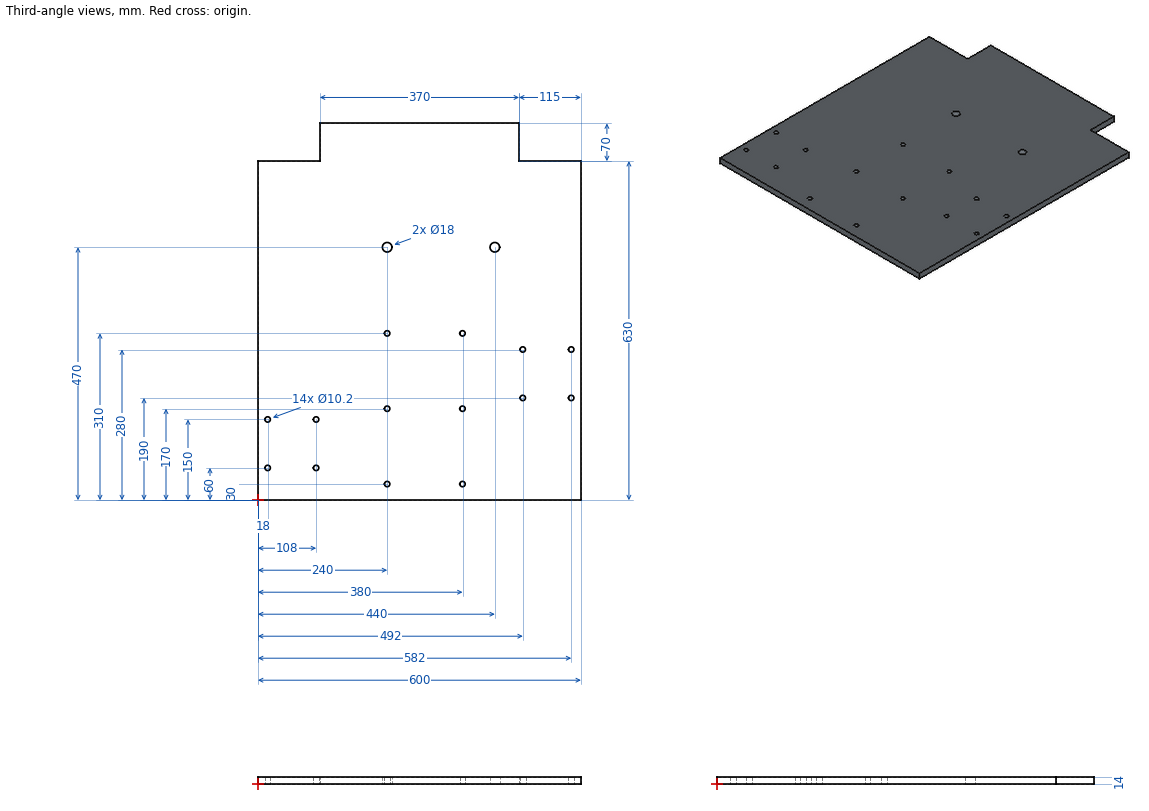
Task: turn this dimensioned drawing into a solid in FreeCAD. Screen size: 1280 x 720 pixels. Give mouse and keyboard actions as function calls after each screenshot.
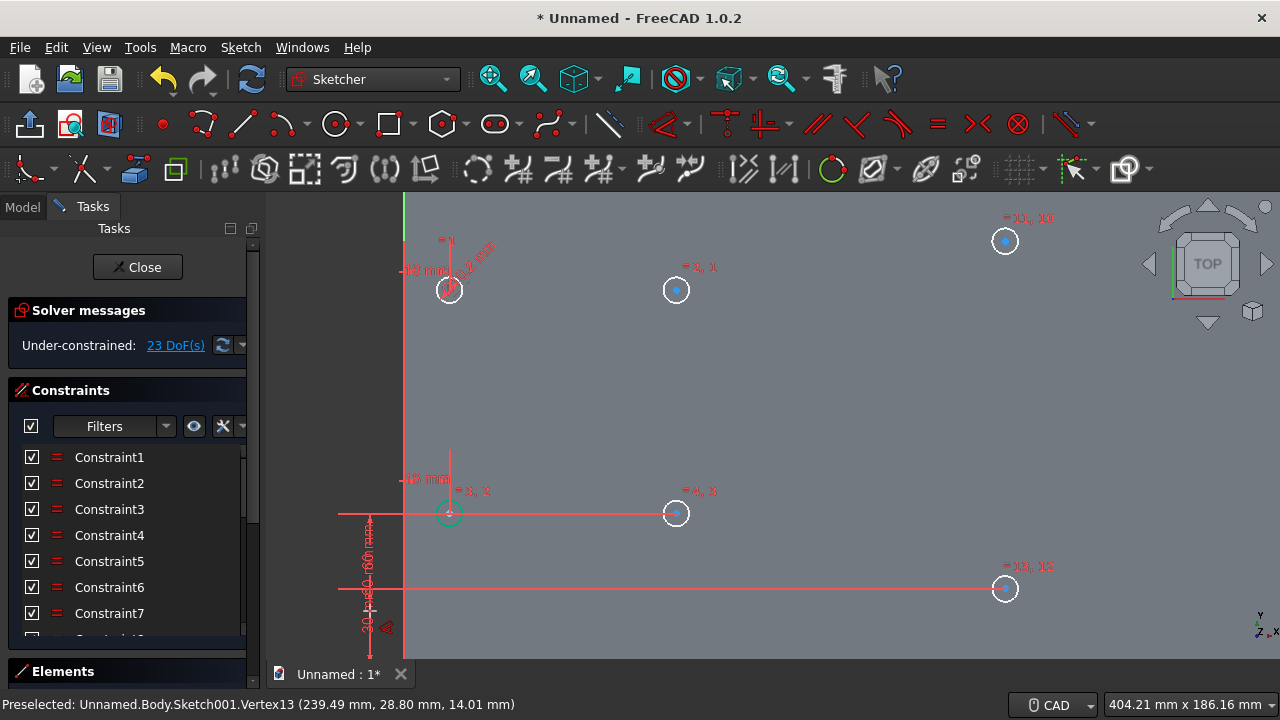
scroll(451, 517, down, 5)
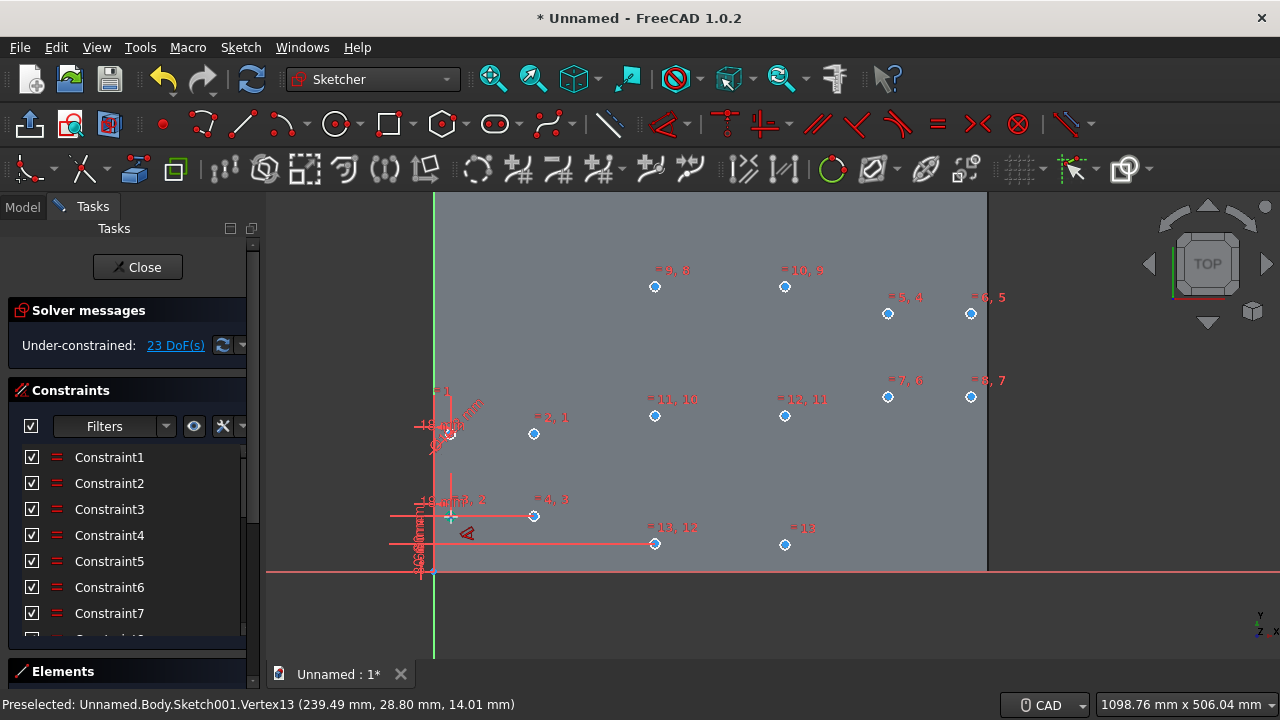
scroll(785, 545, up, 2)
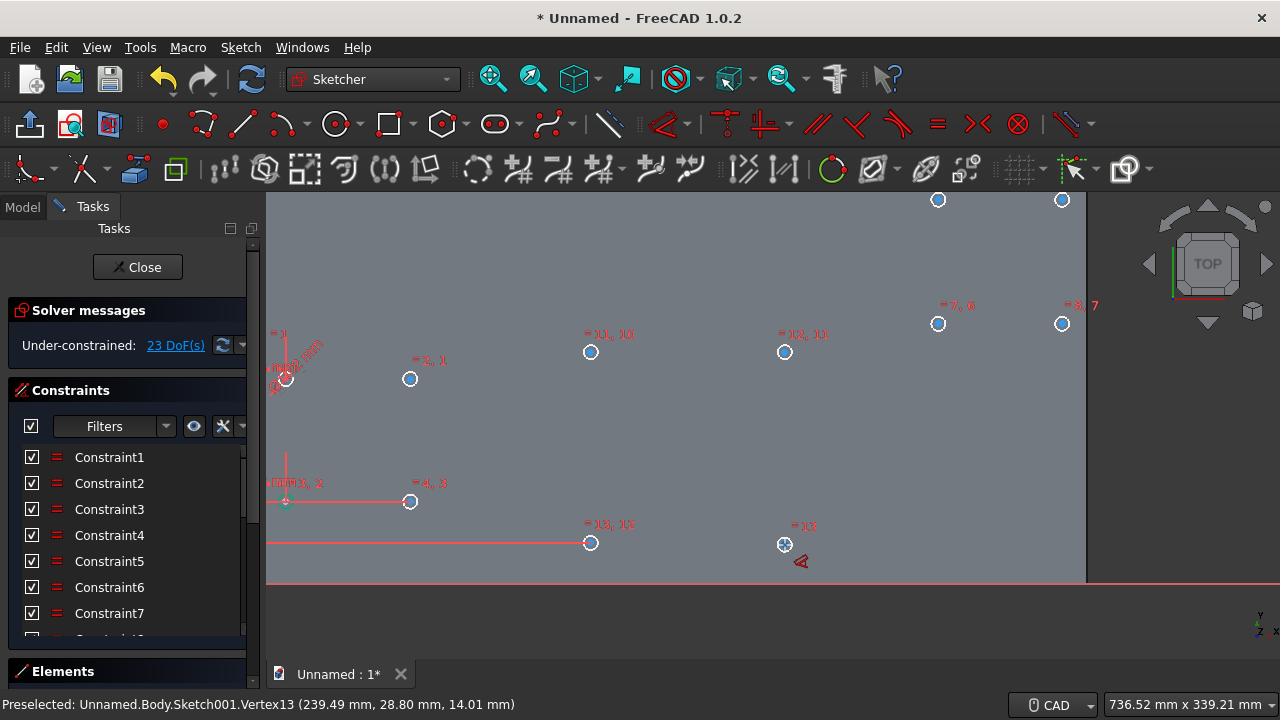
click(785, 545)
click(819, 564)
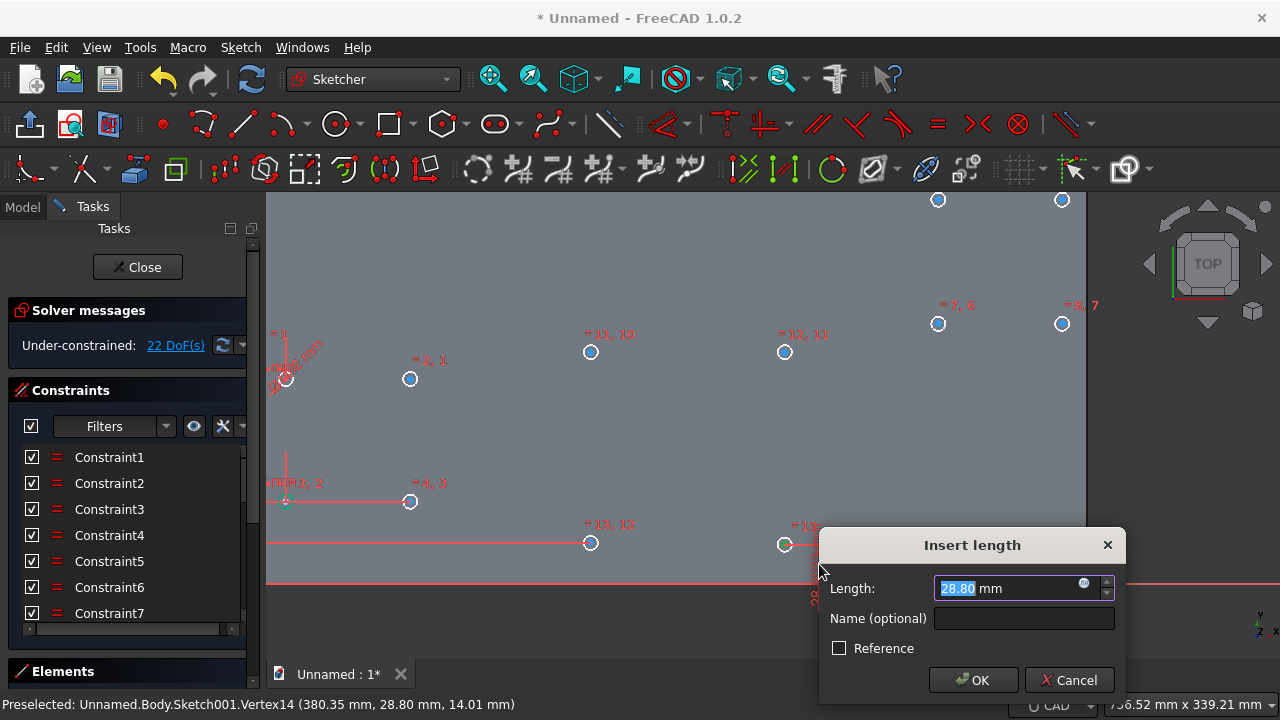
text(30)
key(Return)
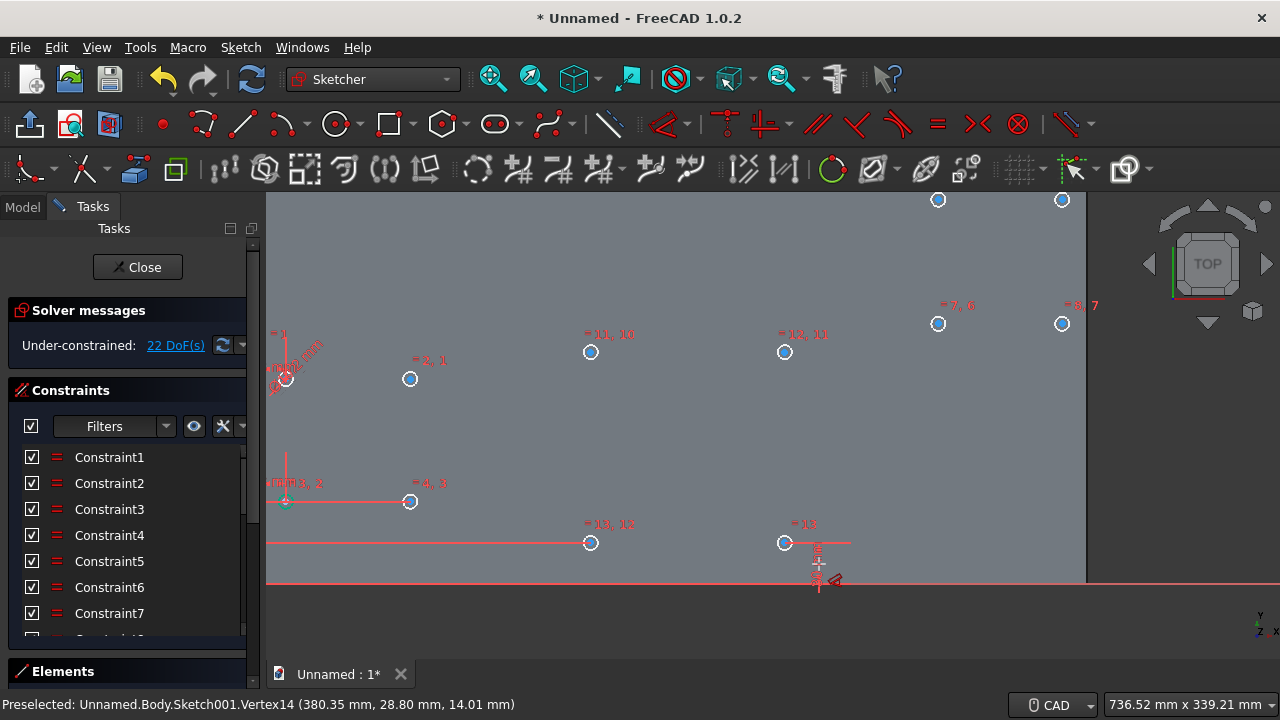
scroll(784, 544, down, 2)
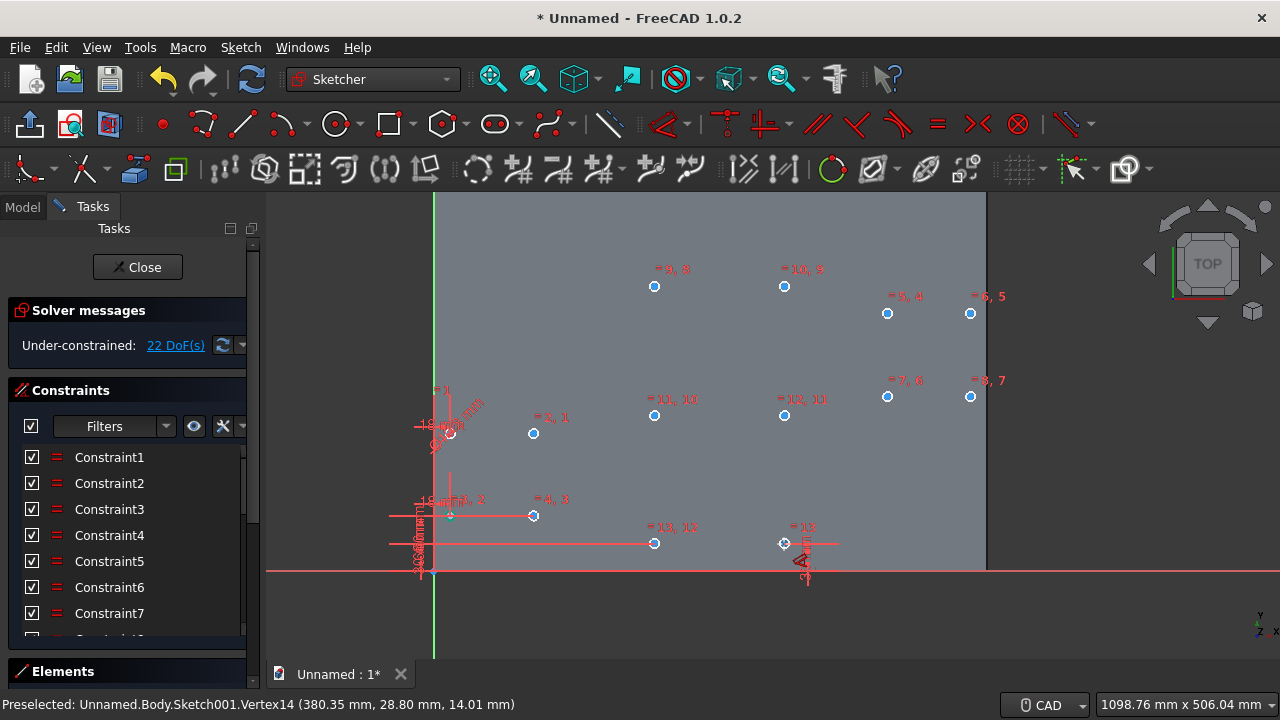
click(450, 434)
click(400, 471)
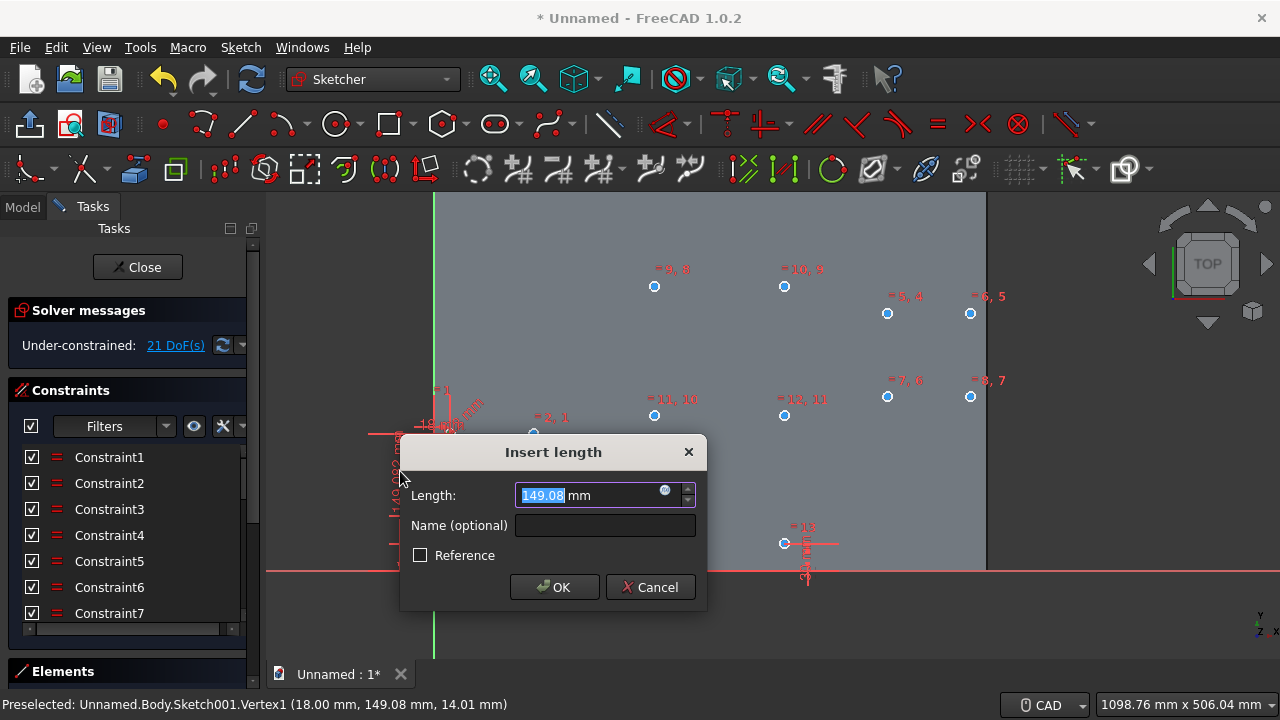
text(150)
key(Return)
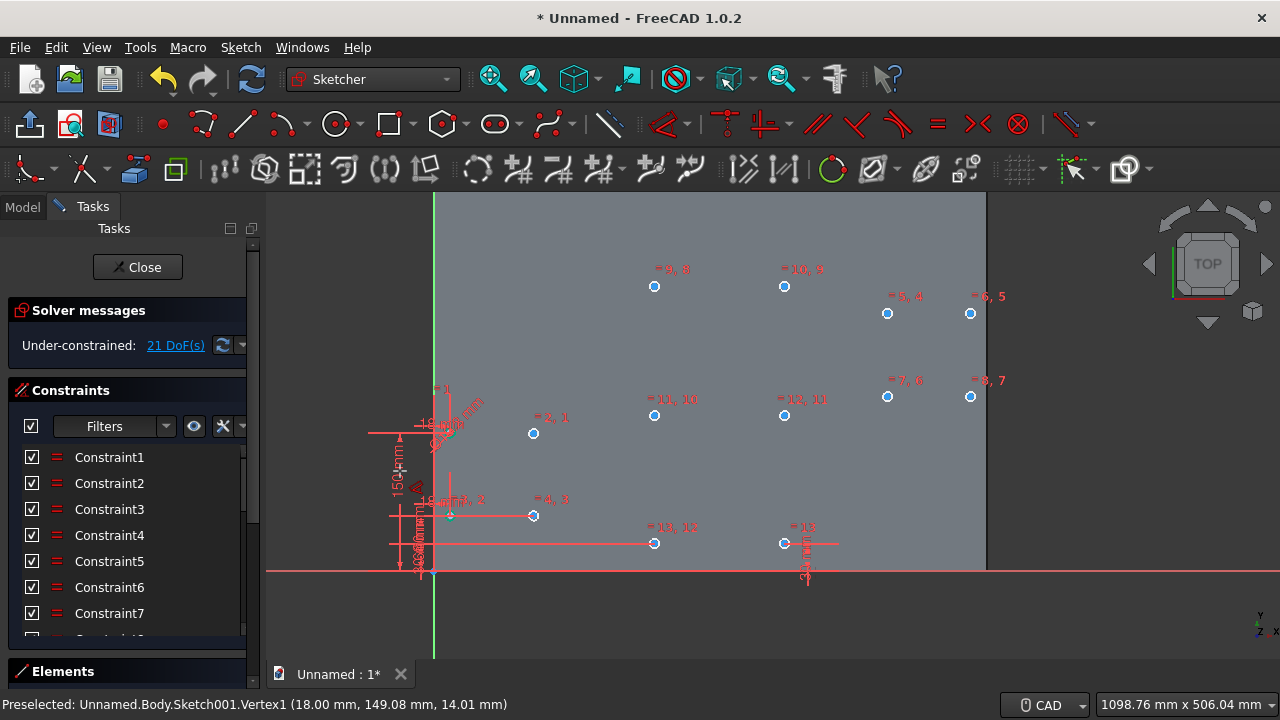
click(534, 434)
click(484, 605)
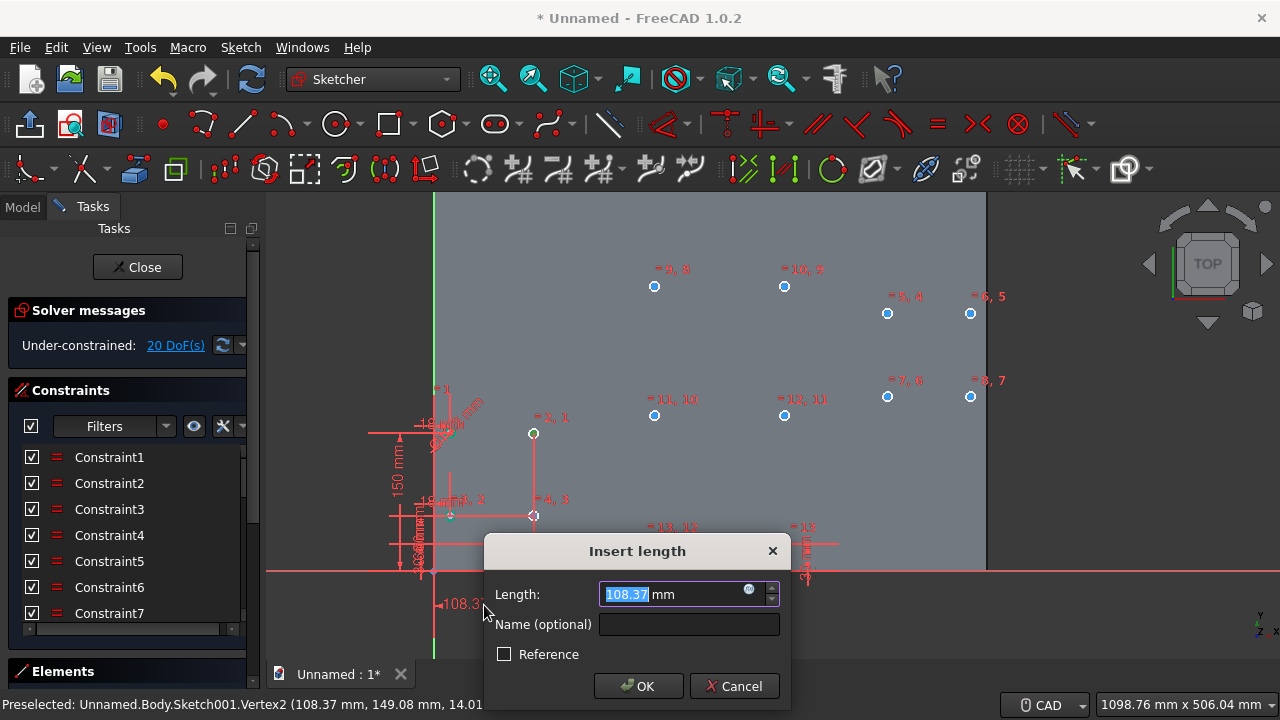
text(108)
key(Return)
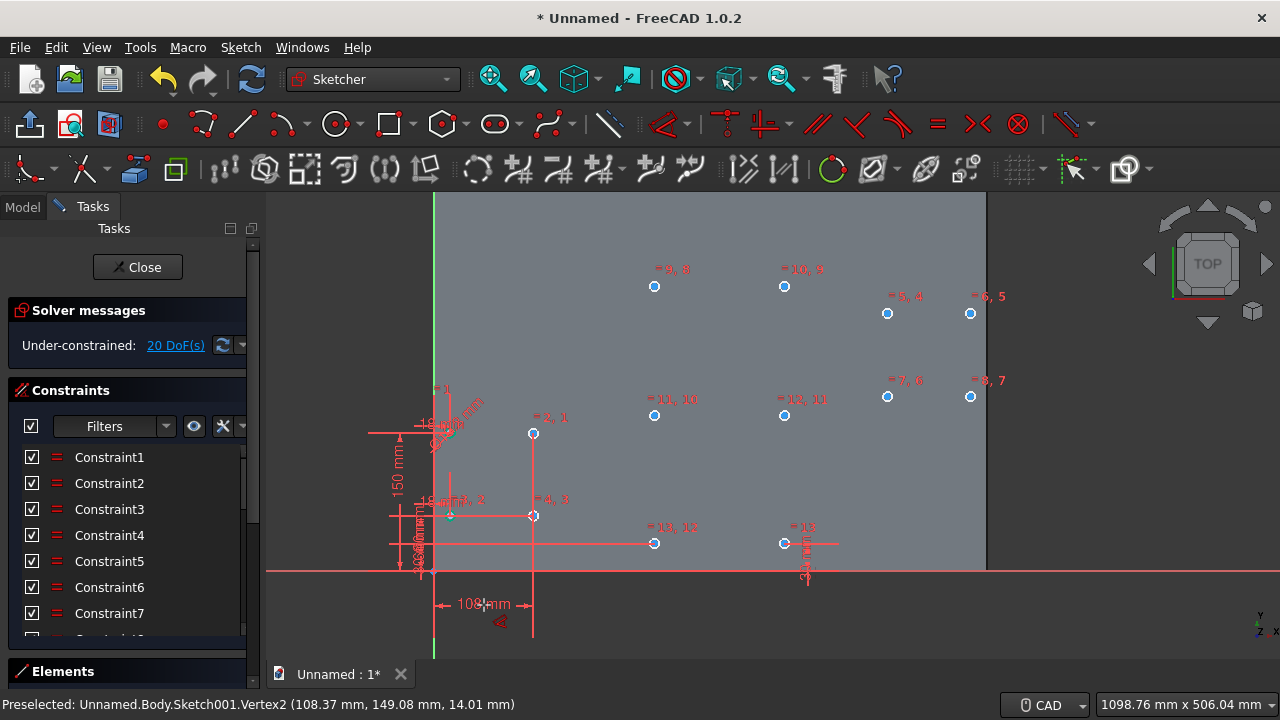
click(533, 434)
click(567, 502)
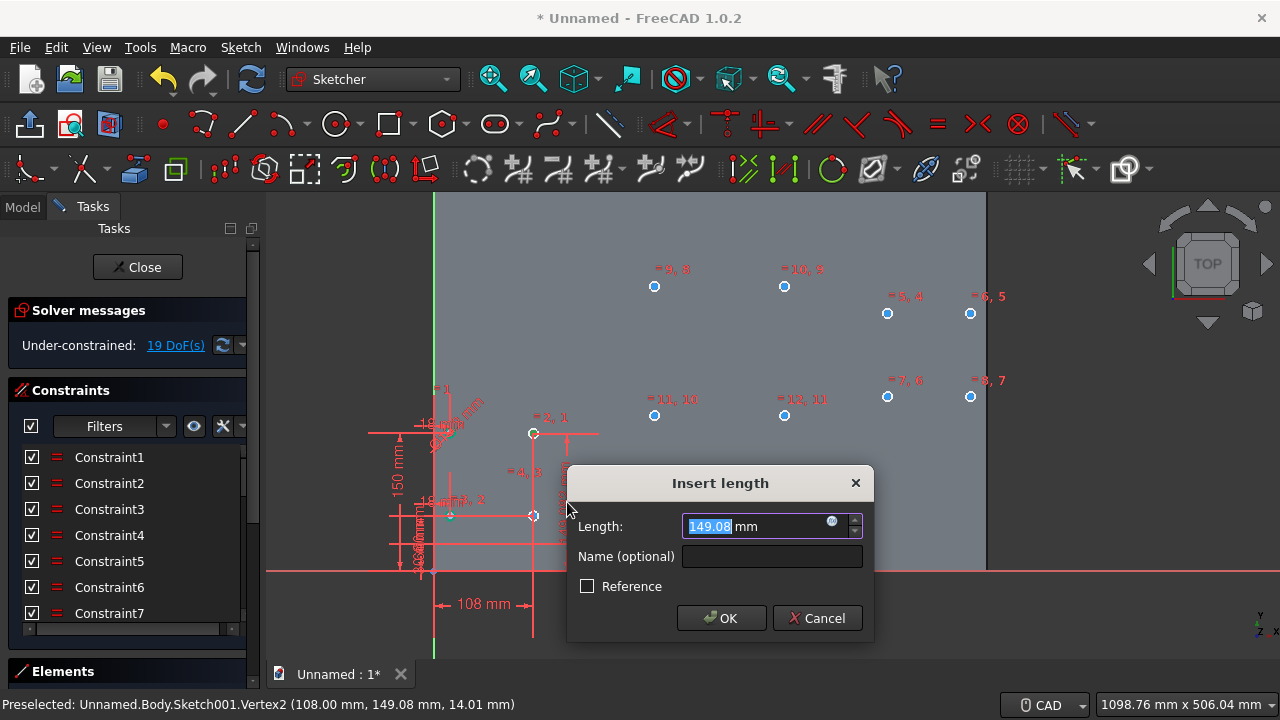
text(150)
key(Return)